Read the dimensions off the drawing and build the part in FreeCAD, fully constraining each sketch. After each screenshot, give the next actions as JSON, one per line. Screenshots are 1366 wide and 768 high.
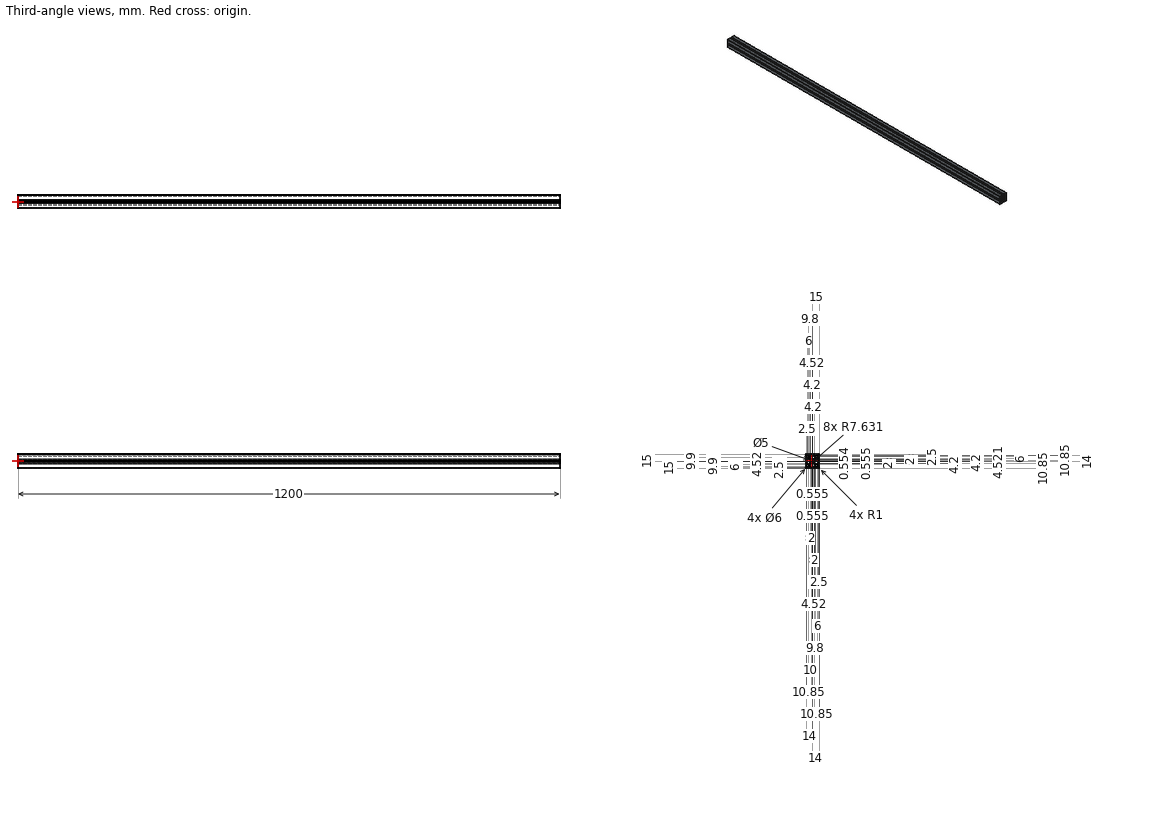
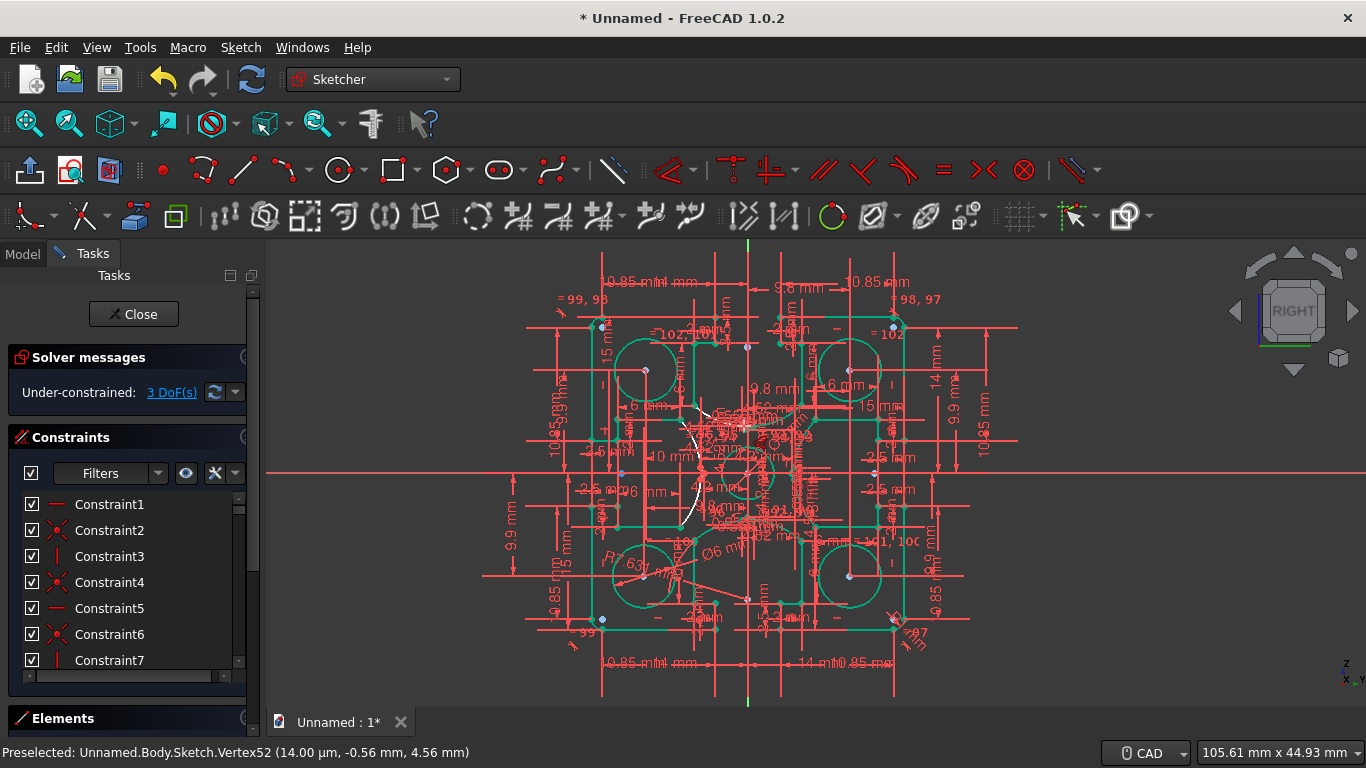
{"action": "scroll", "coordinate": [742, 426], "scroll_direction": "up", "scroll_amount": 3}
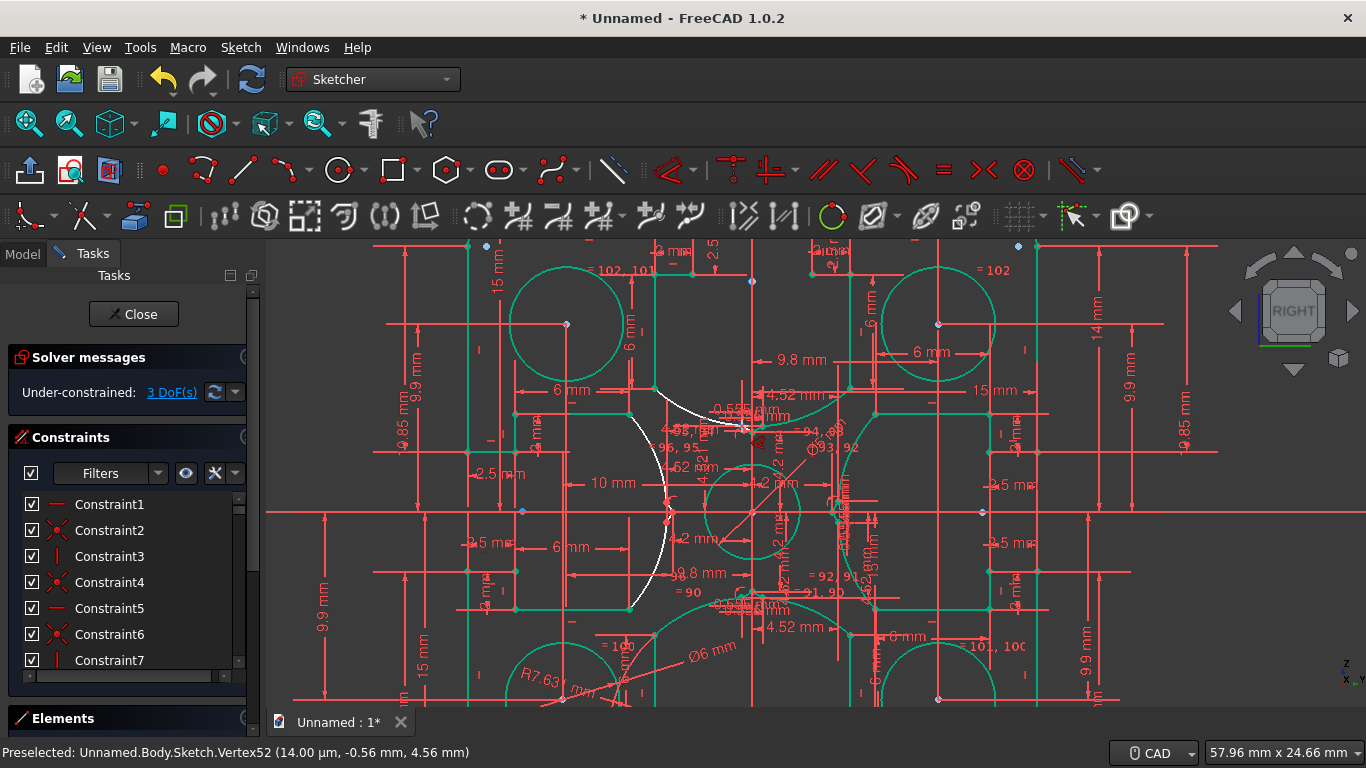
{"action": "left_click", "coordinate": [742, 426]}
{"action": "left_click", "coordinate": [858, 469]}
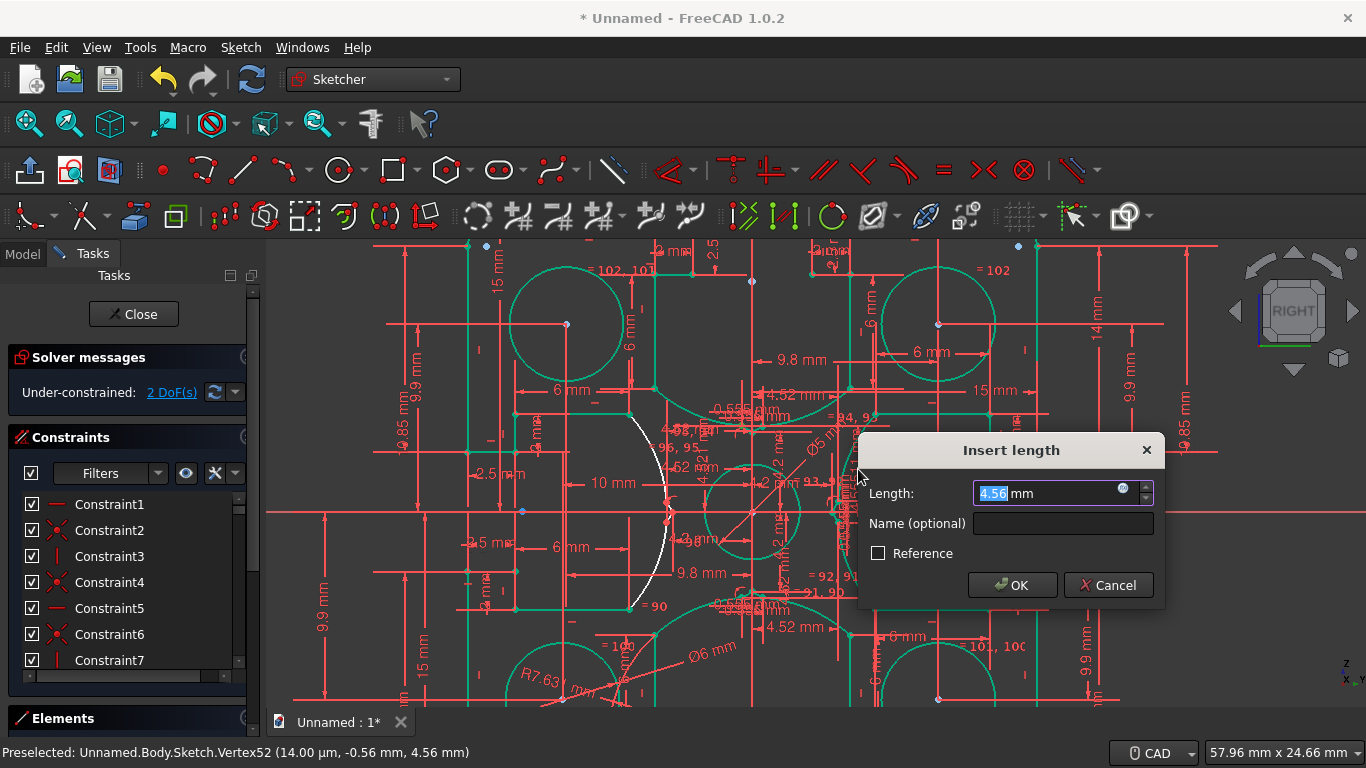
{"action": "type", "text": "4.521"}
{"action": "key", "text": "Return"}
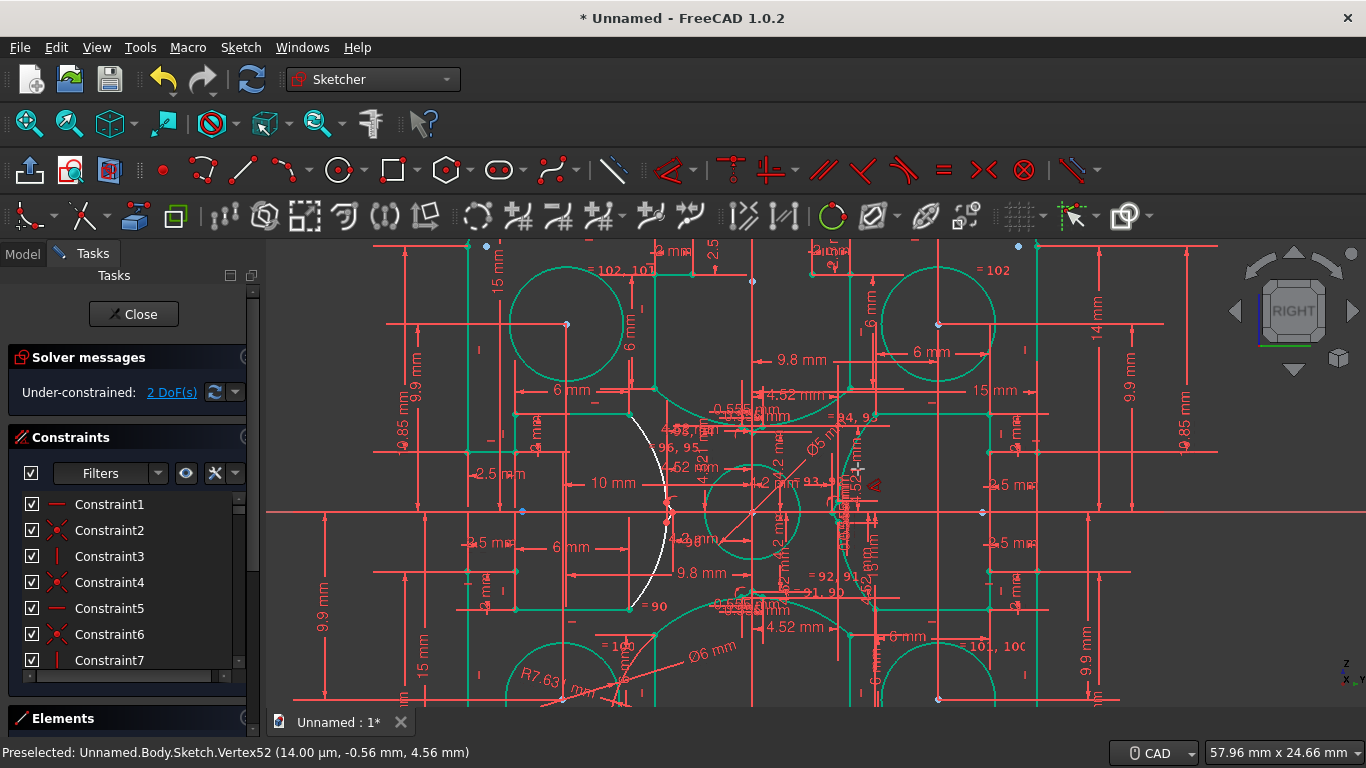
{"action": "scroll", "coordinate": [667, 502], "scroll_direction": "up", "scroll_amount": 7}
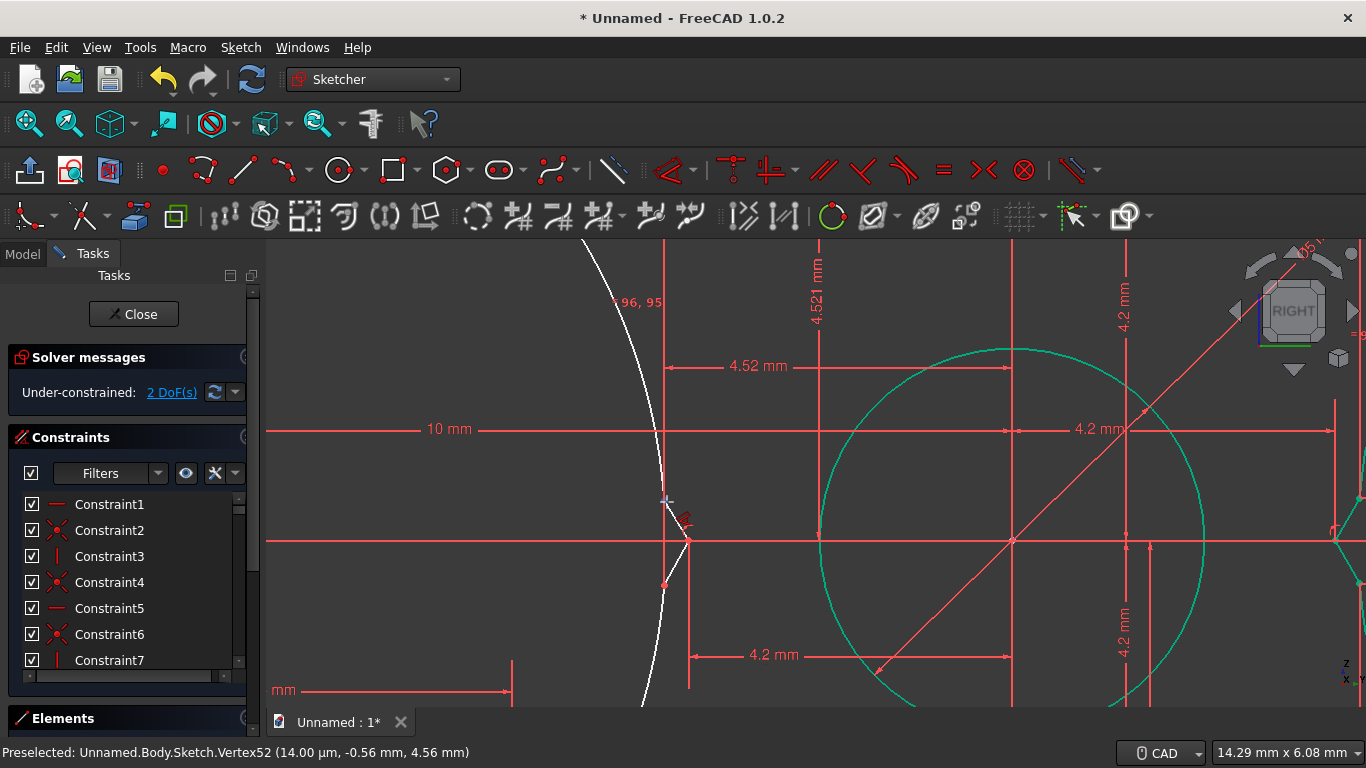
{"action": "left_click", "coordinate": [664, 501]}
{"action": "left_click", "coordinate": [630, 521]}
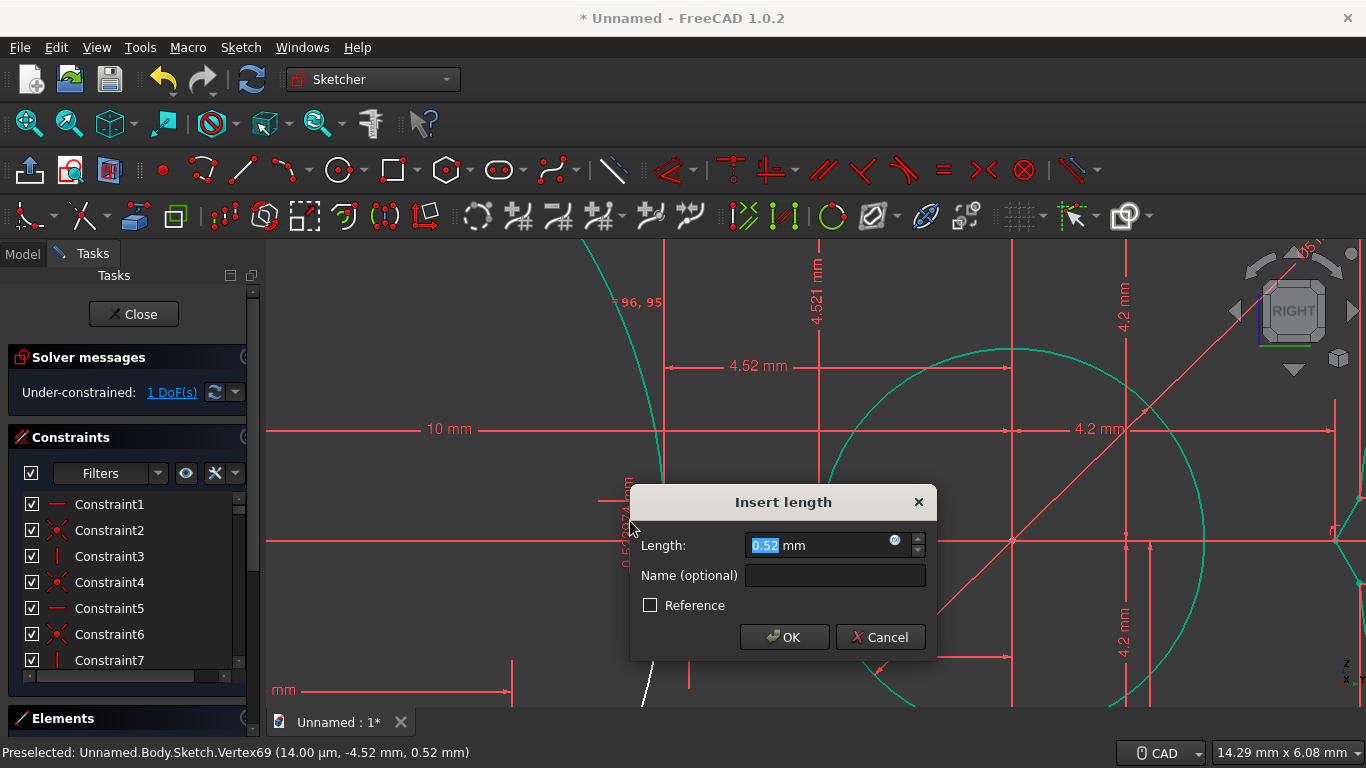
{"action": "type", "text": "0.555"}
{"action": "key", "text": "Return"}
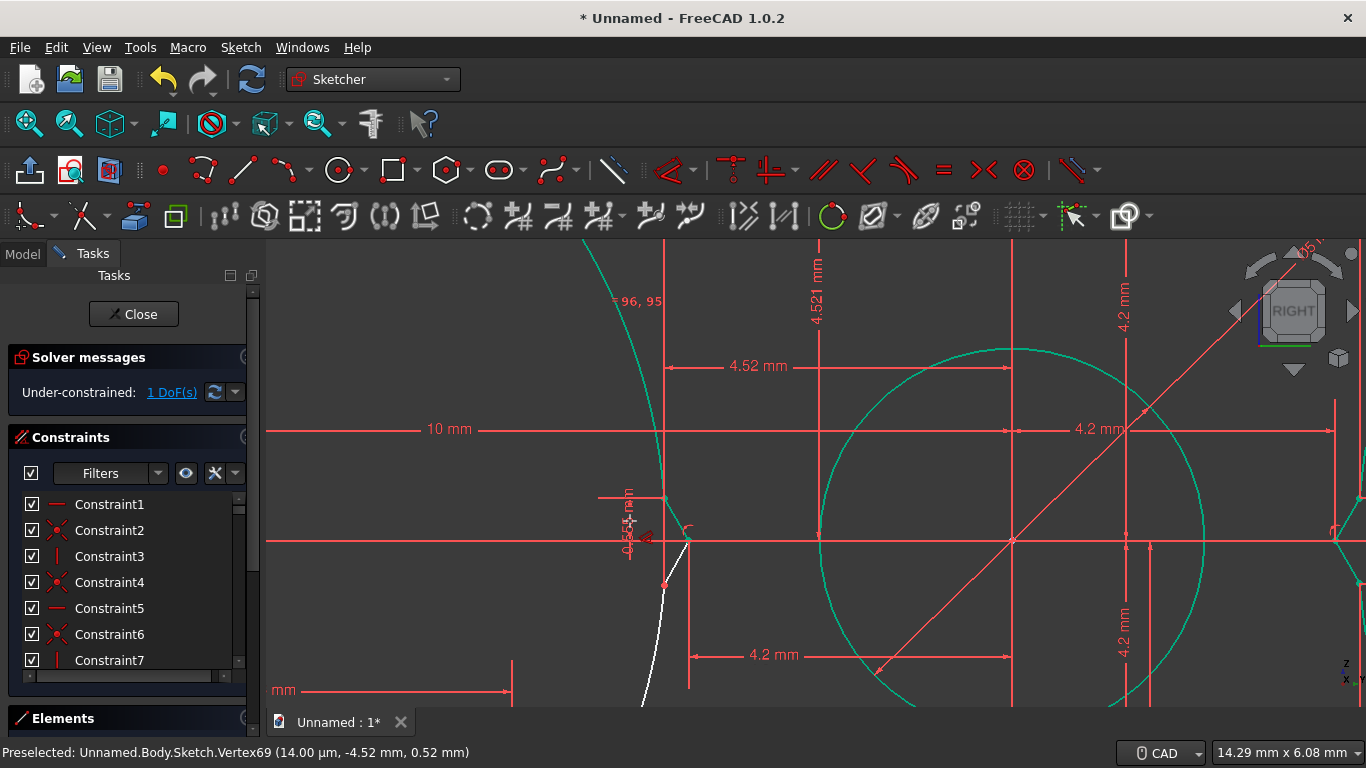
{"action": "left_click", "coordinate": [664, 585]}
{"action": "left_click", "coordinate": [630, 563]}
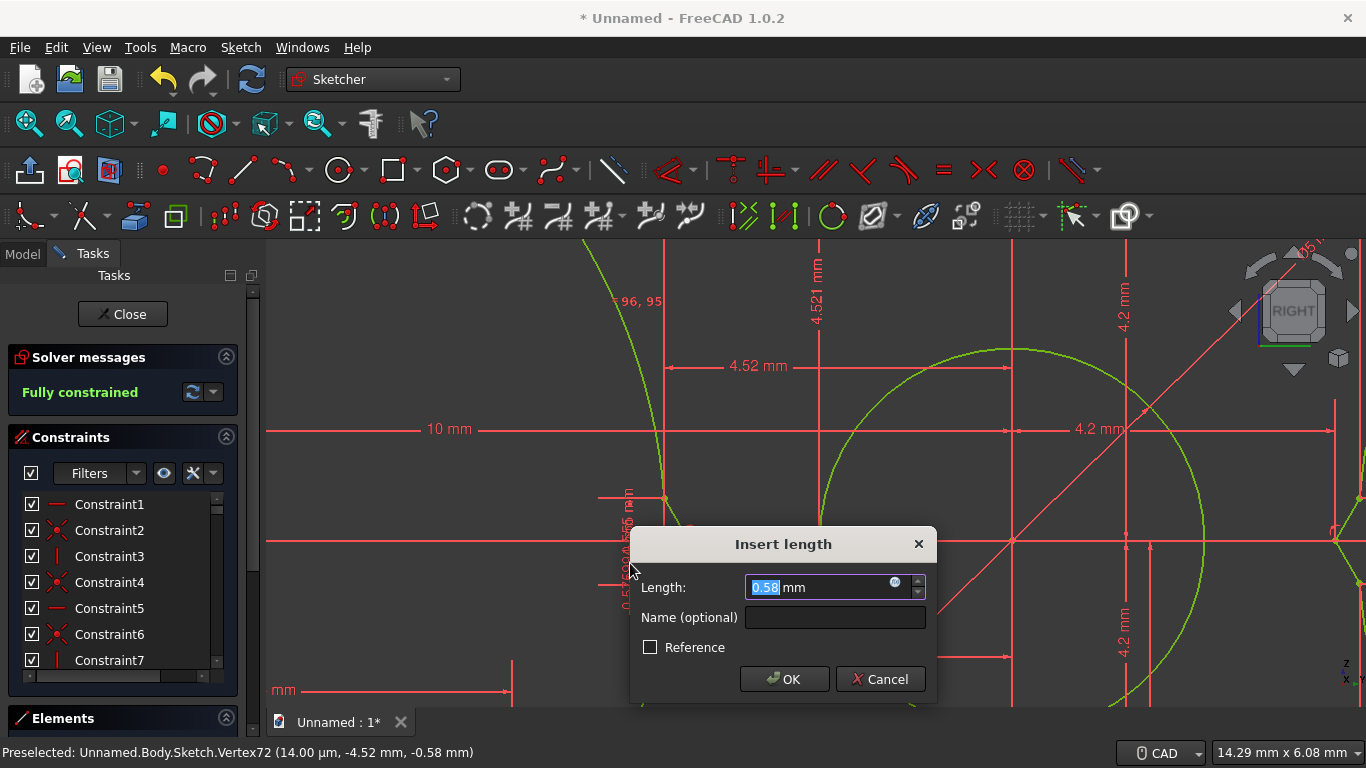
{"action": "type", "text": "0.554"}
{"action": "key", "text": "Return"}
{"action": "key", "text": "Escape"}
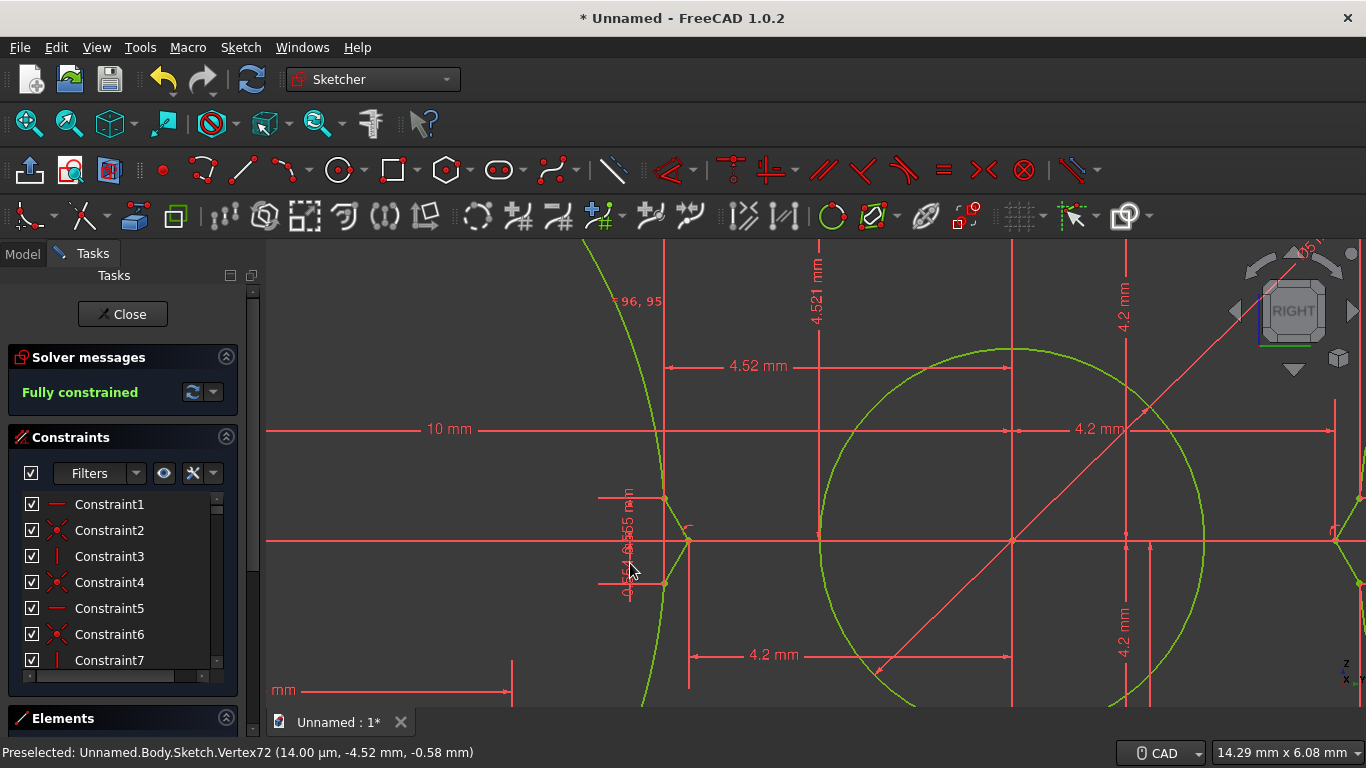
{"action": "left_click", "coordinate": [123, 314]}